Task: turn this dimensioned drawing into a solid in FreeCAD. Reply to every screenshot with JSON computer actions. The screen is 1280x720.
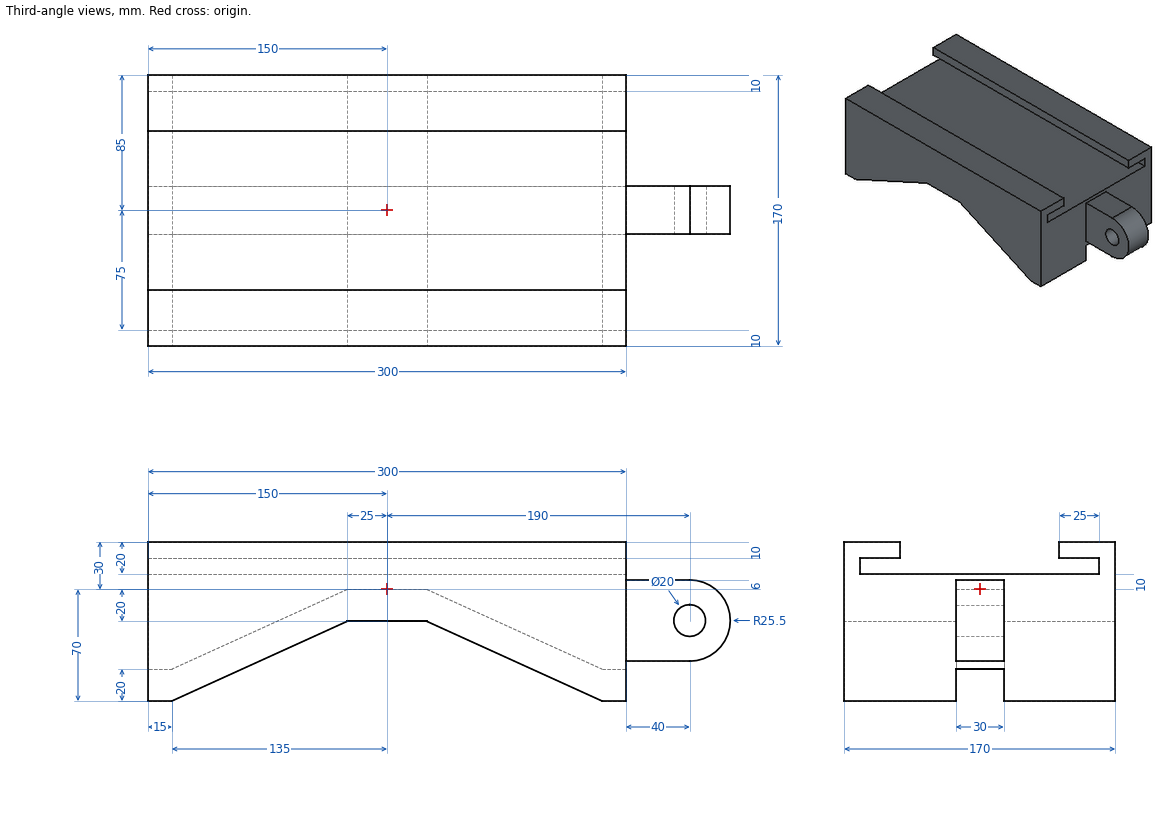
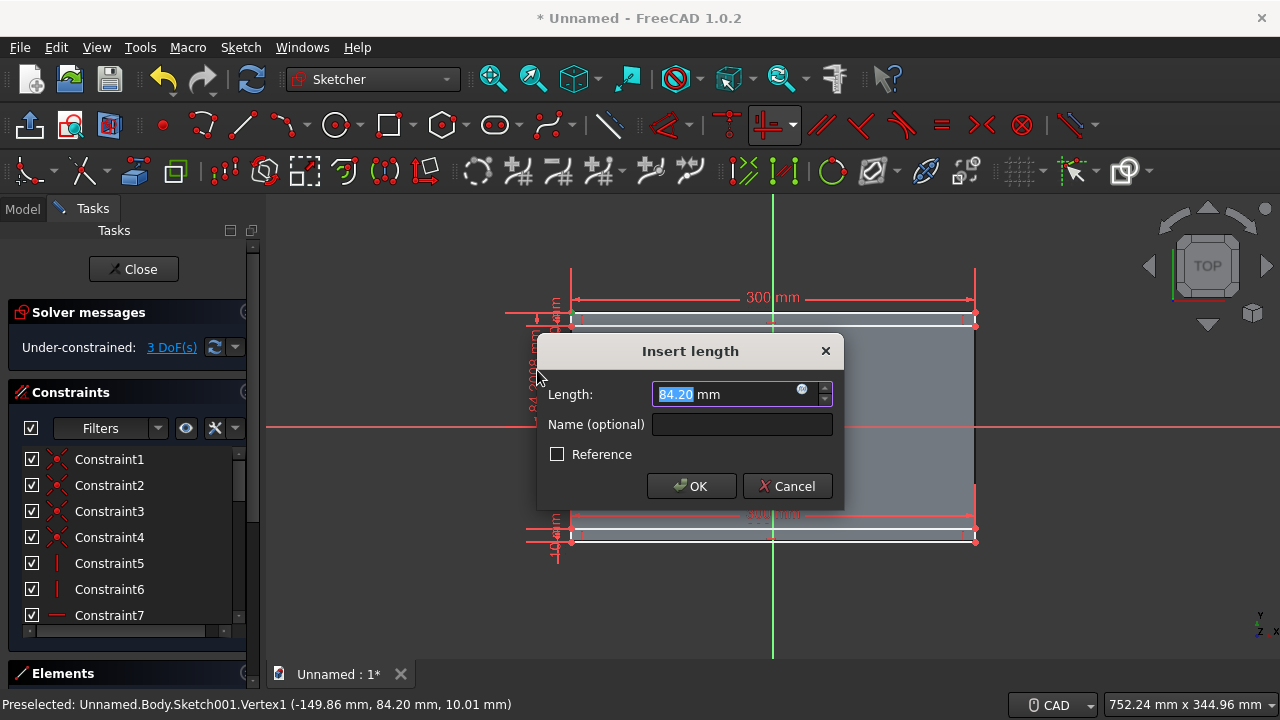
{"action": "type", "text": "85"}
{"action": "key", "text": "Return"}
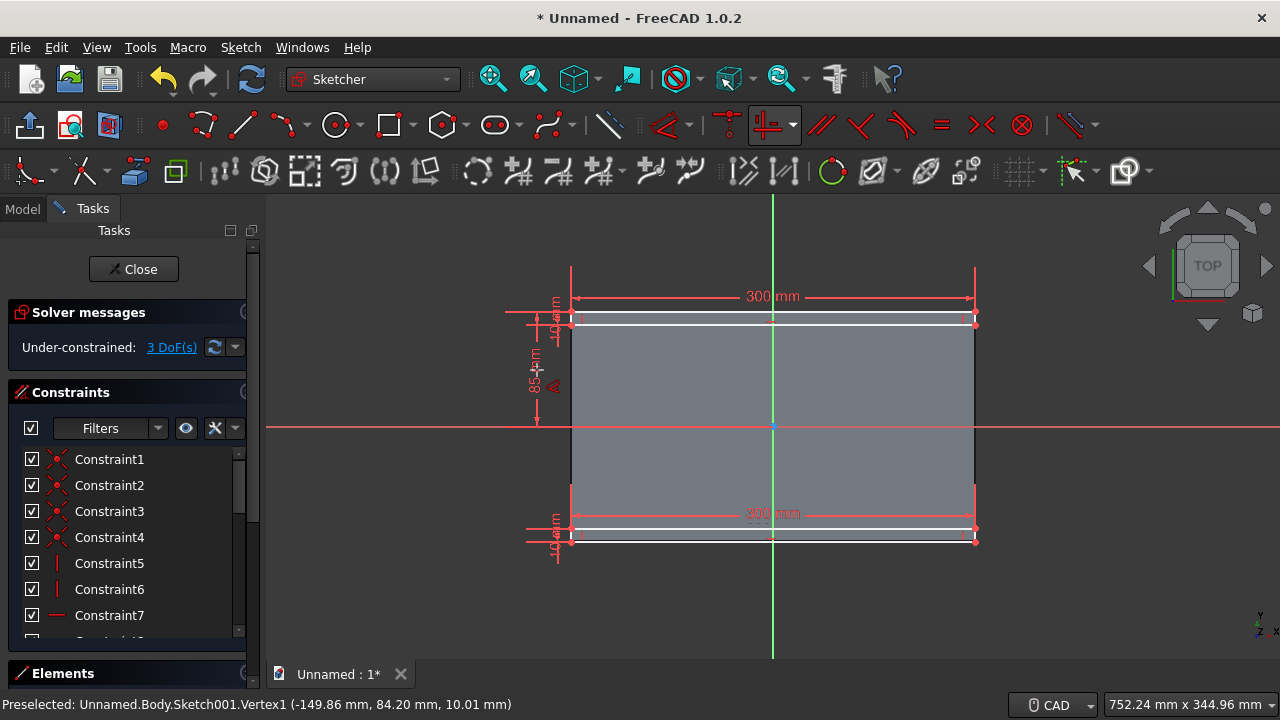
{"action": "left_click", "coordinate": [571, 529]}
{"action": "left_click", "coordinate": [537, 478]}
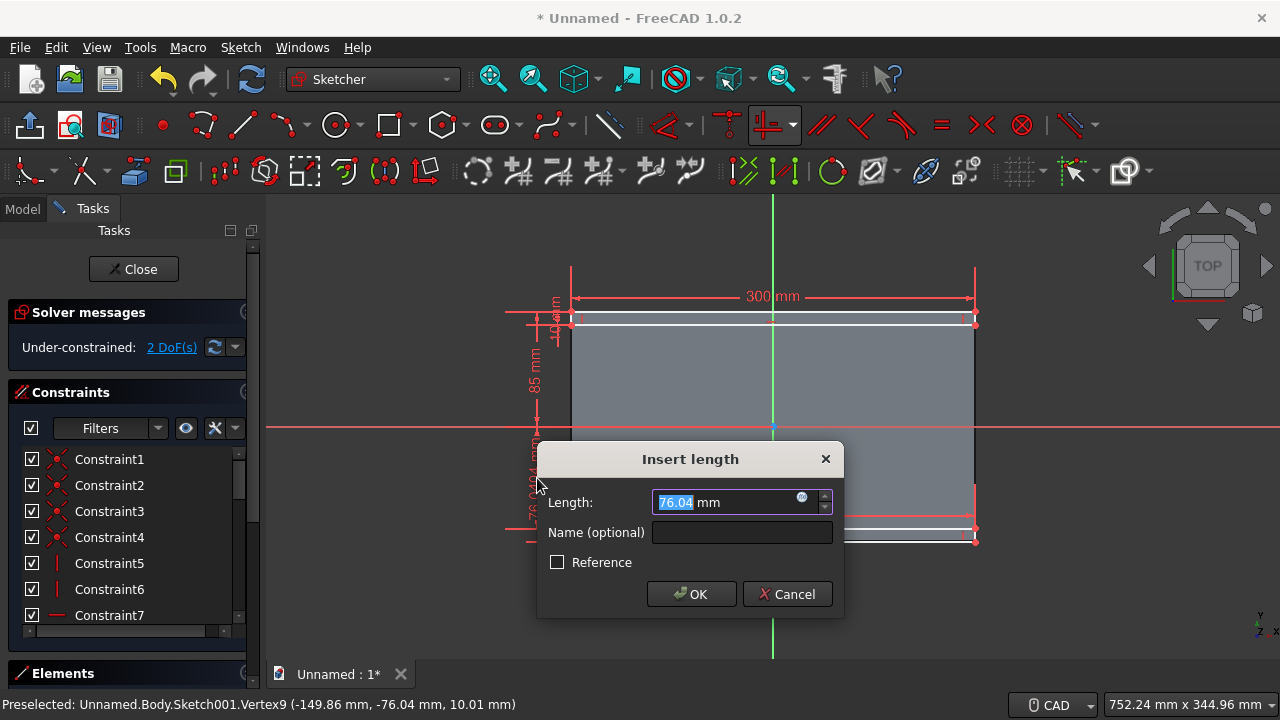
{"action": "type", "text": "75"}
{"action": "key", "text": "Return"}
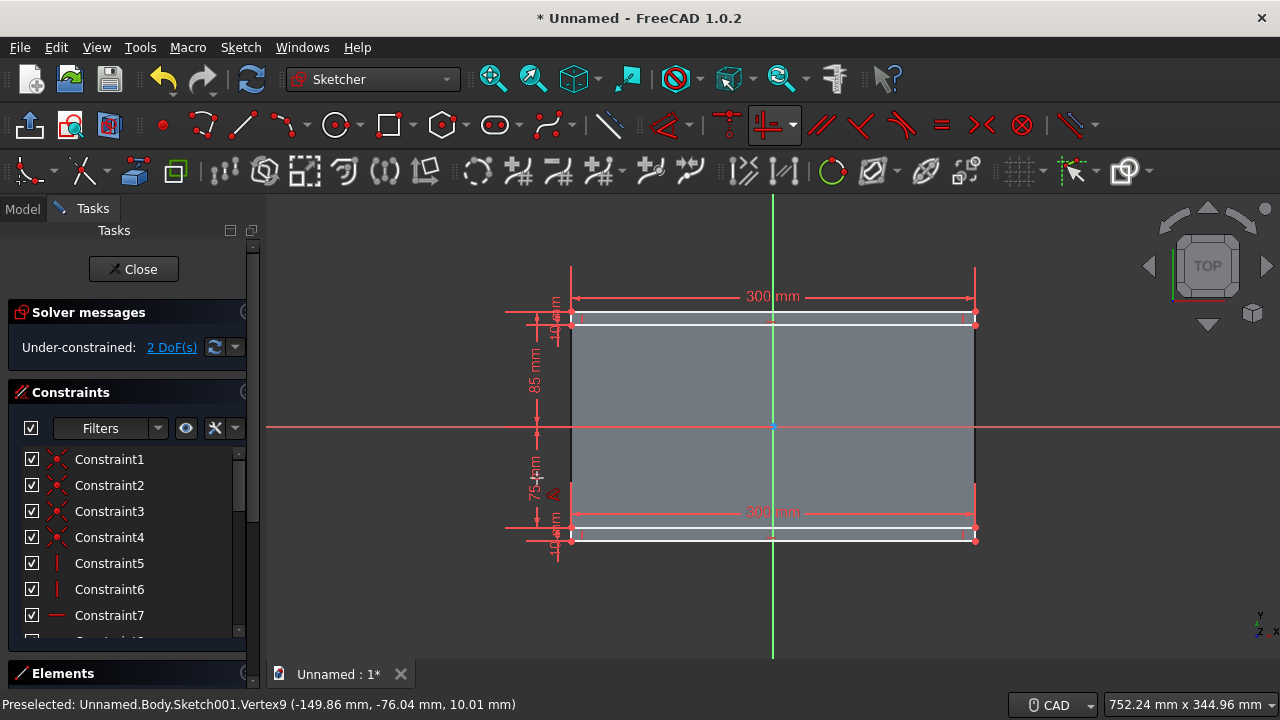
{"action": "left_click", "coordinate": [571, 312]}
{"action": "left_click", "coordinate": [672, 278]}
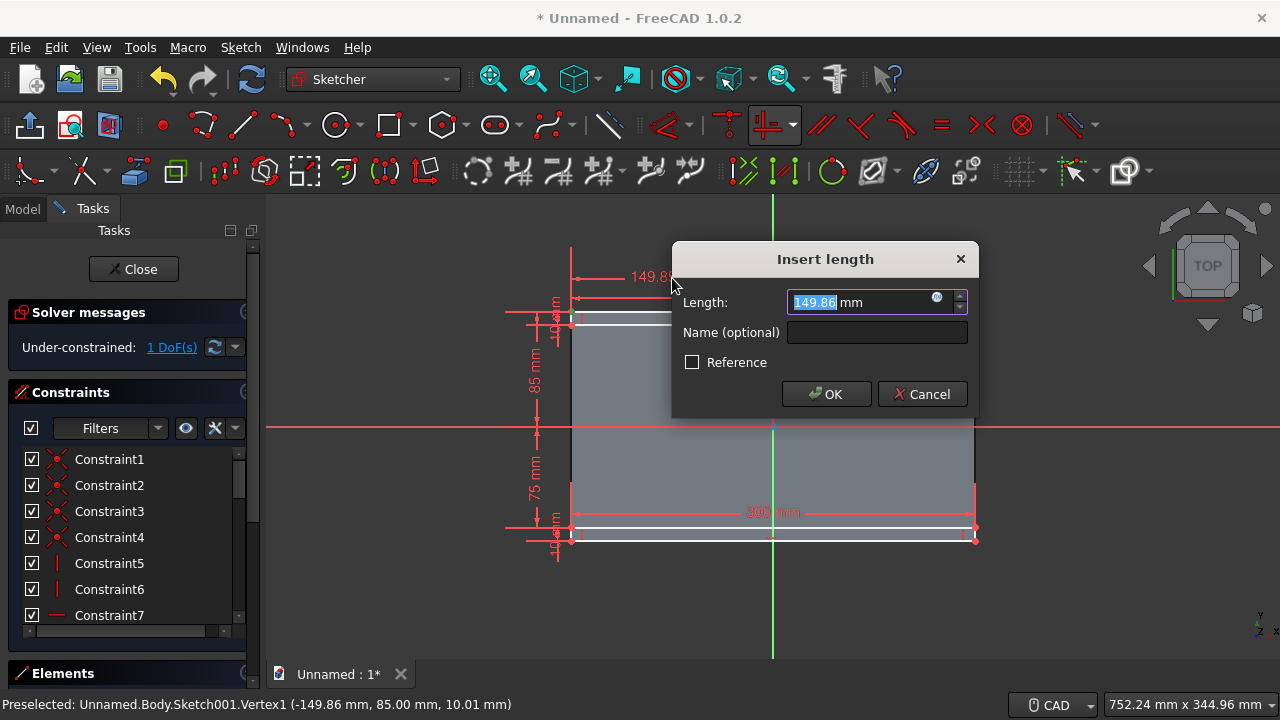
{"action": "type", "text": "150"}
{"action": "key", "text": "Return"}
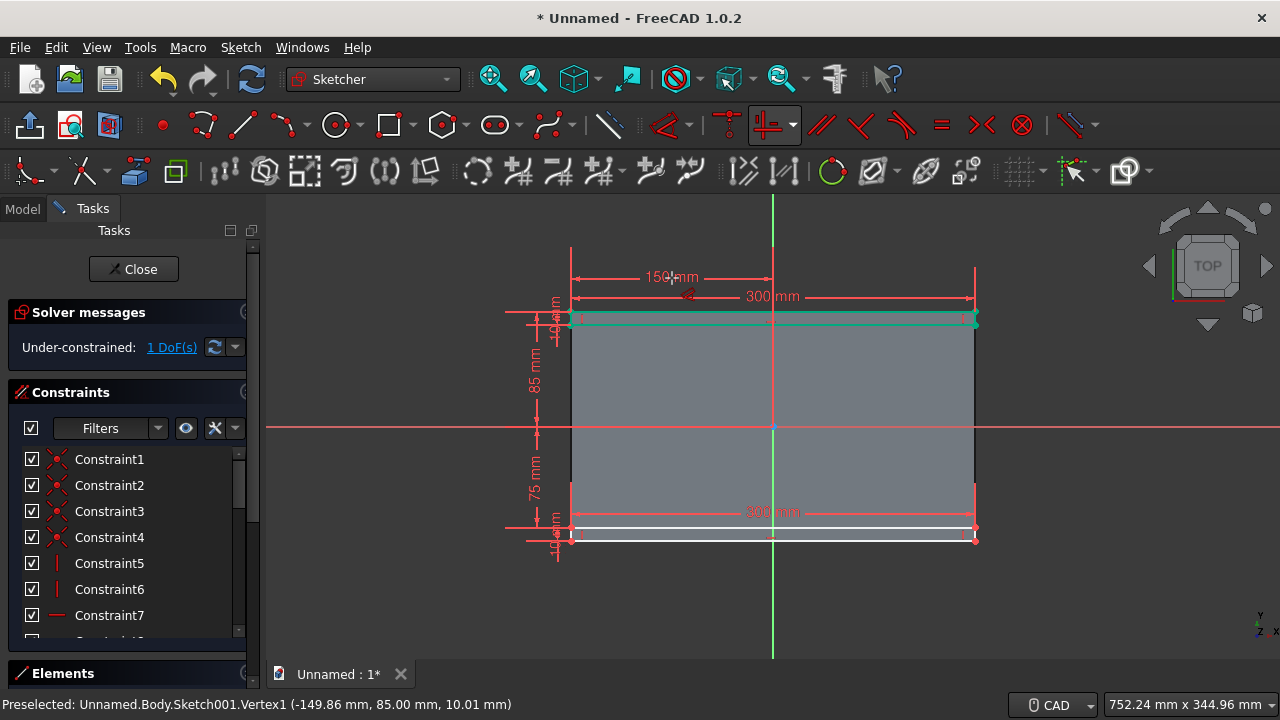
{"action": "left_click", "coordinate": [571, 528]}
{"action": "left_click", "coordinate": [672, 562]}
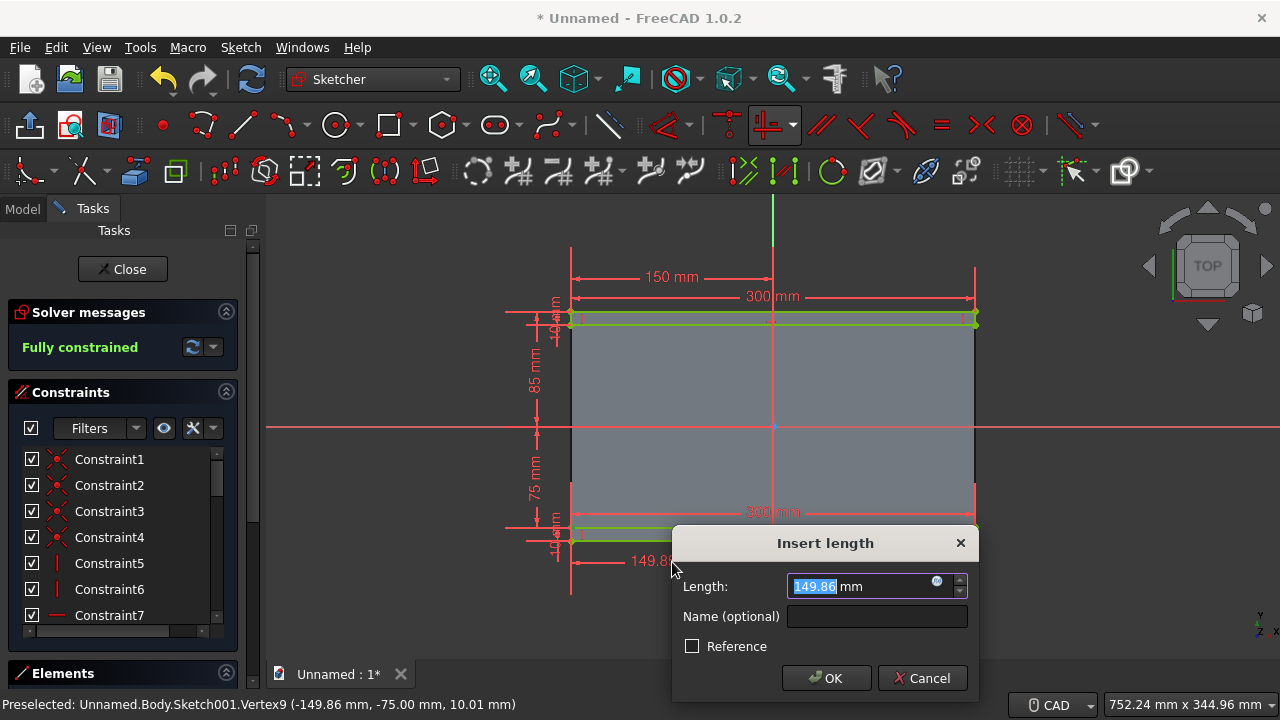
{"action": "type", "text": "150"}
{"action": "key", "text": "Return"}
{"action": "key", "text": "Escape"}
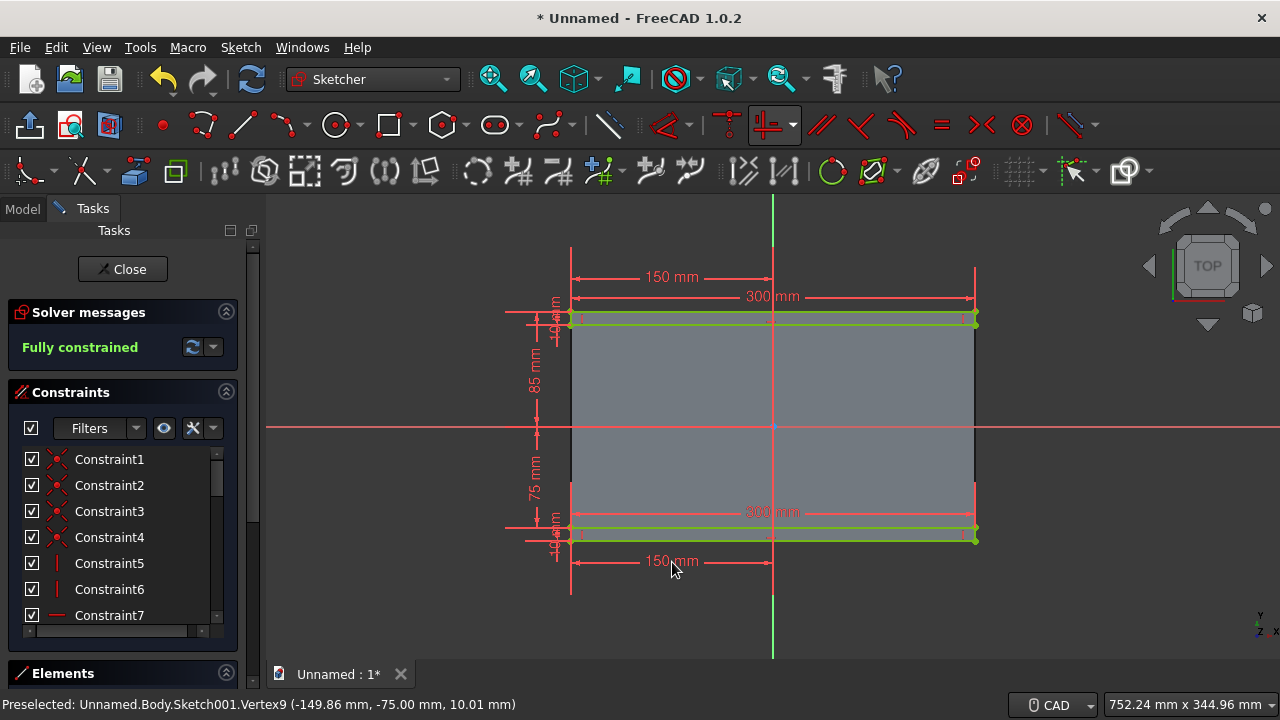
{"action": "left_click", "coordinate": [123, 269]}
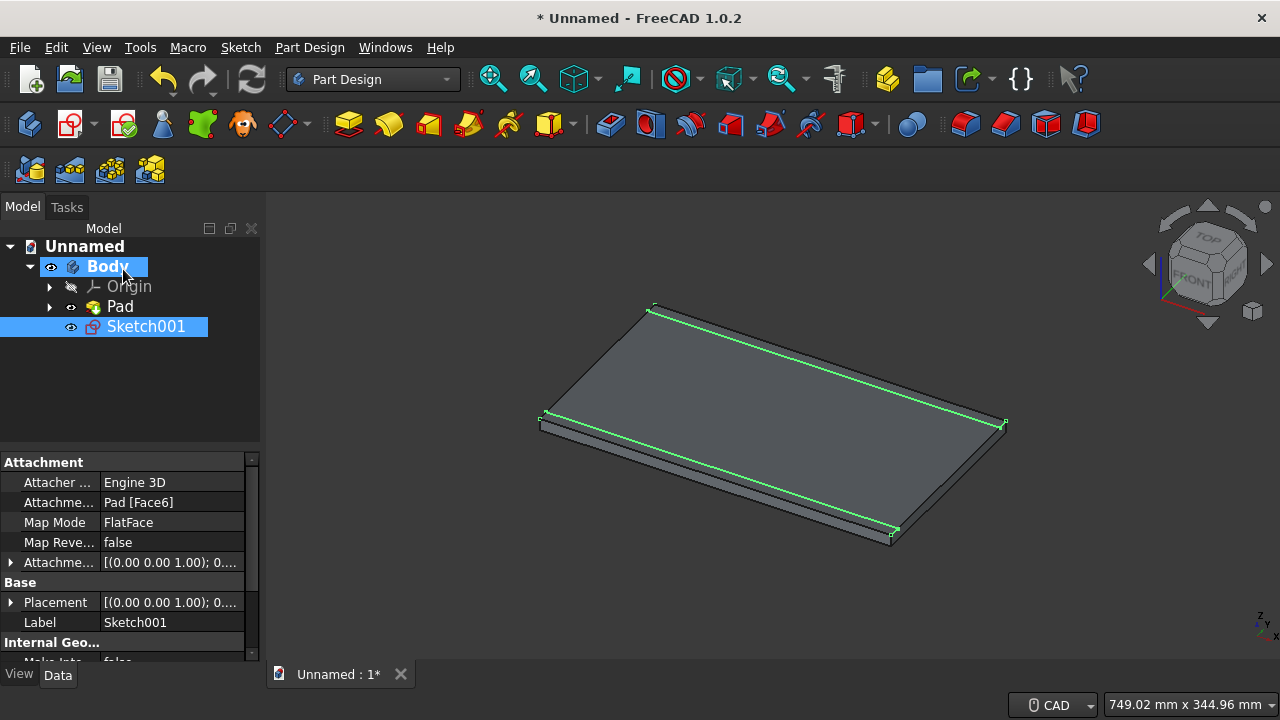
{"action": "left_click", "coordinate": [350, 124]}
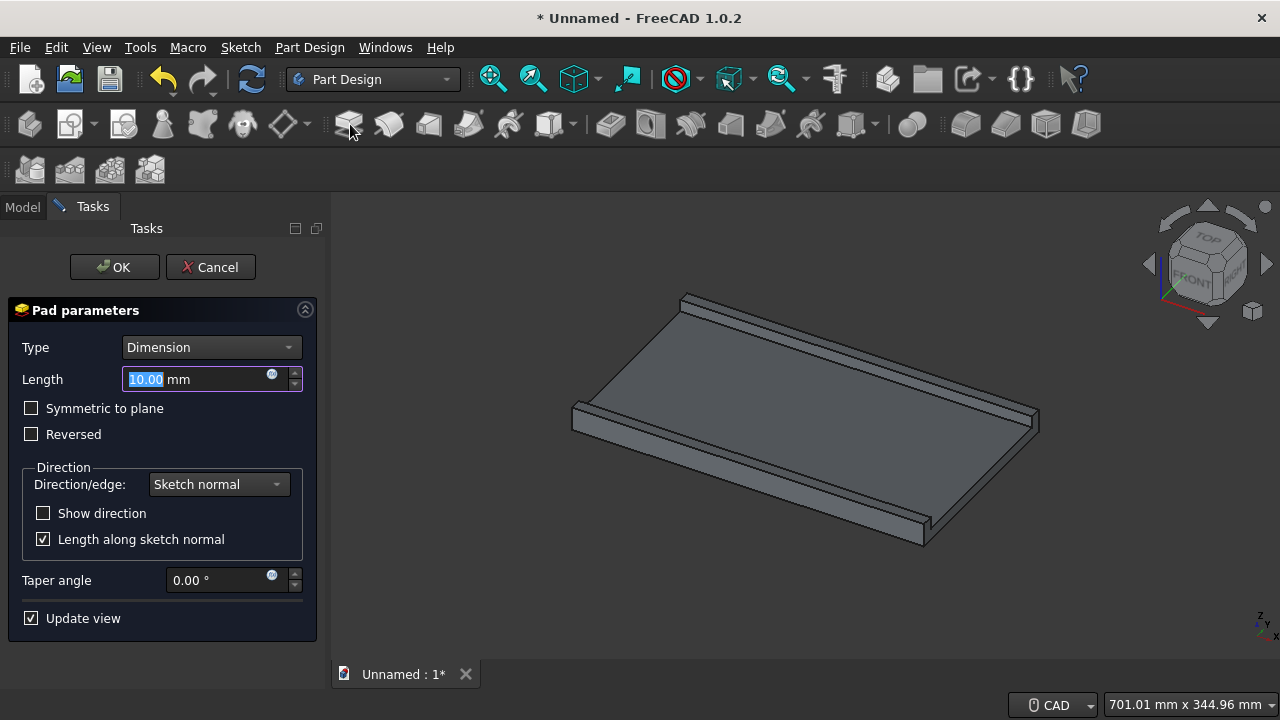
{"action": "type", "text": "20"}
{"action": "key", "text": "Tab"}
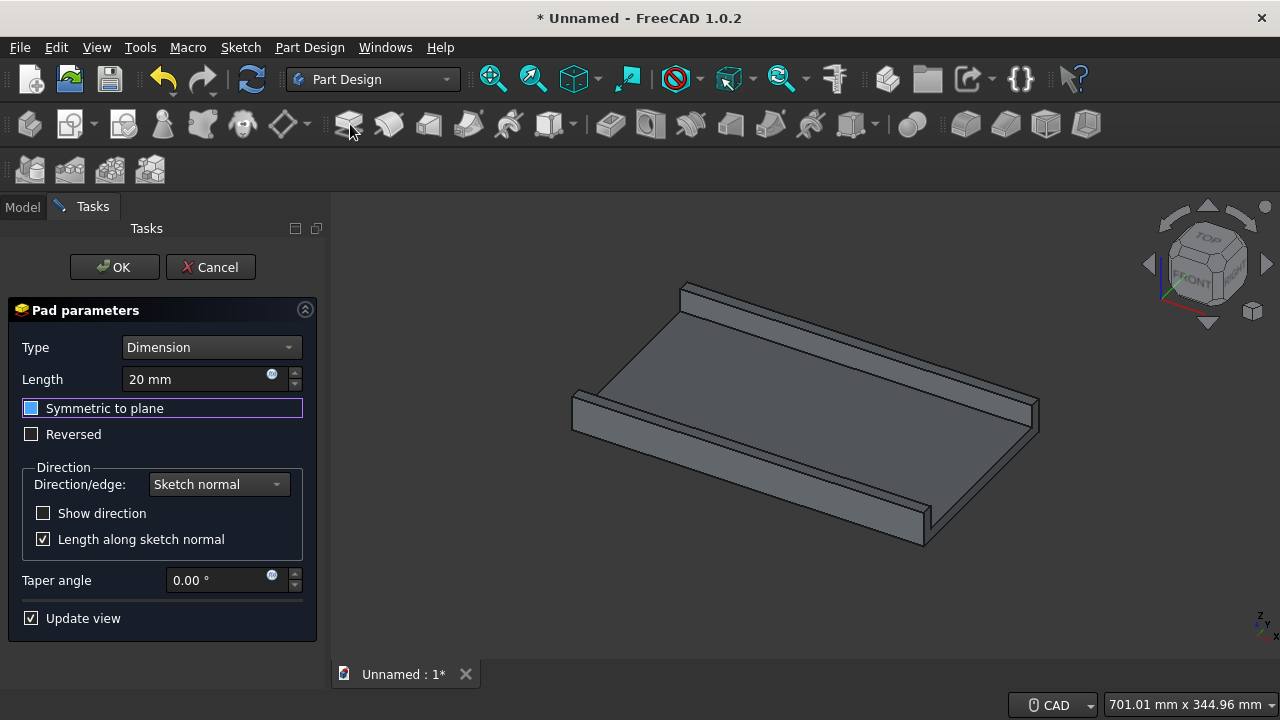
{"action": "left_click", "coordinate": [115, 267]}